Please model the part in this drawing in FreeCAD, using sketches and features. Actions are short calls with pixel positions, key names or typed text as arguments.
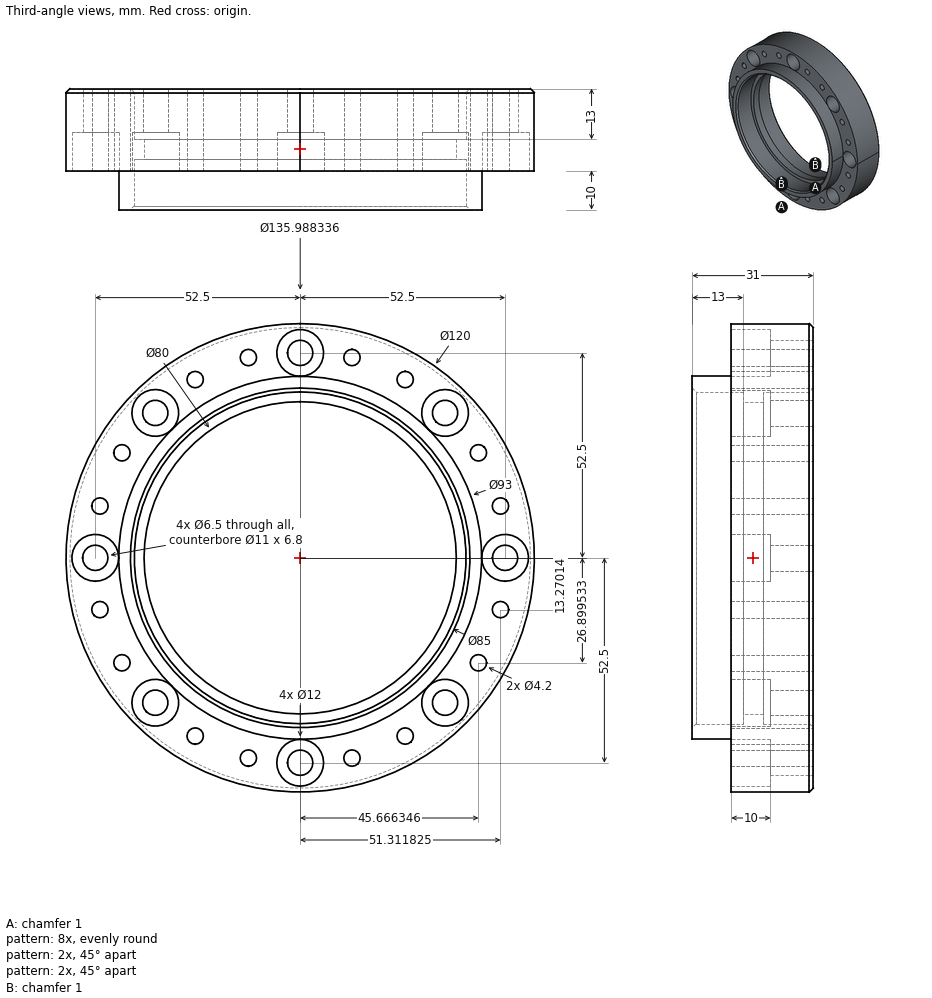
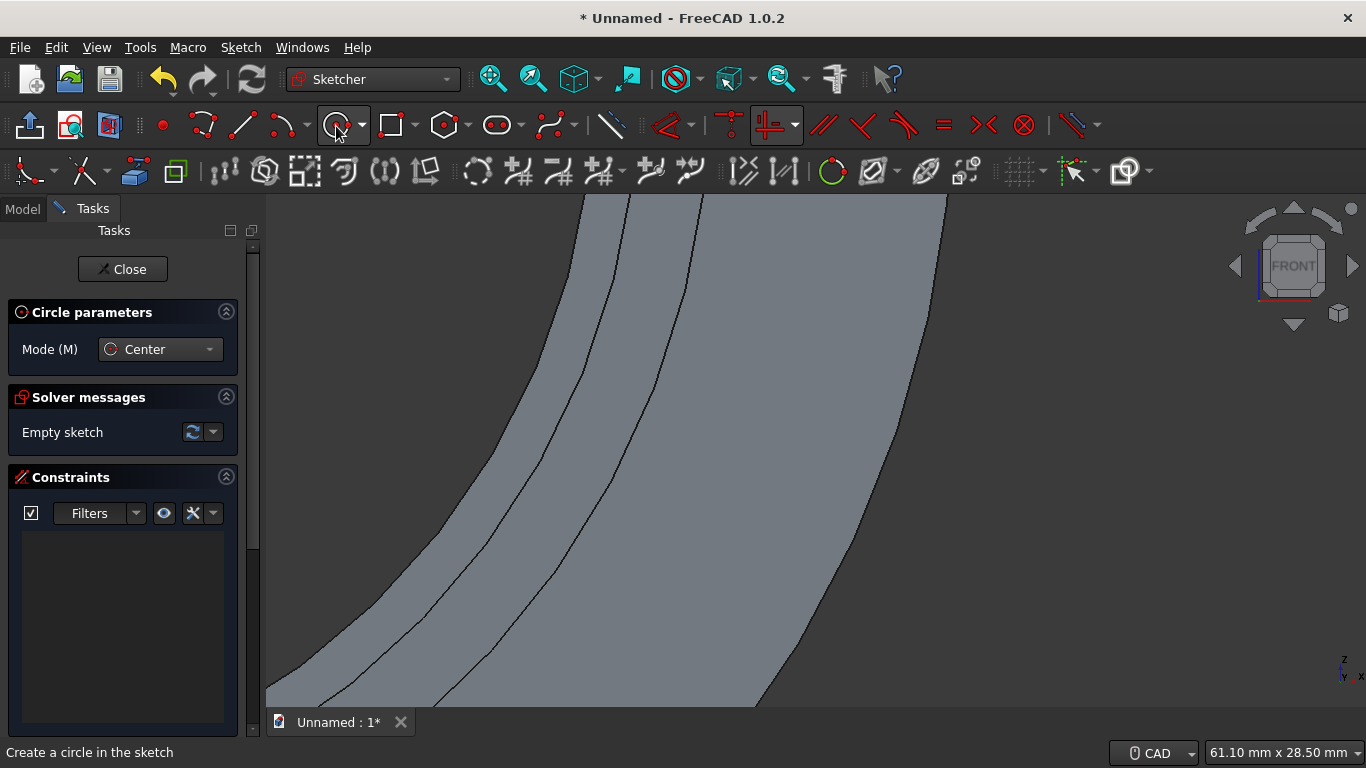
click(695, 570)
move(722, 544)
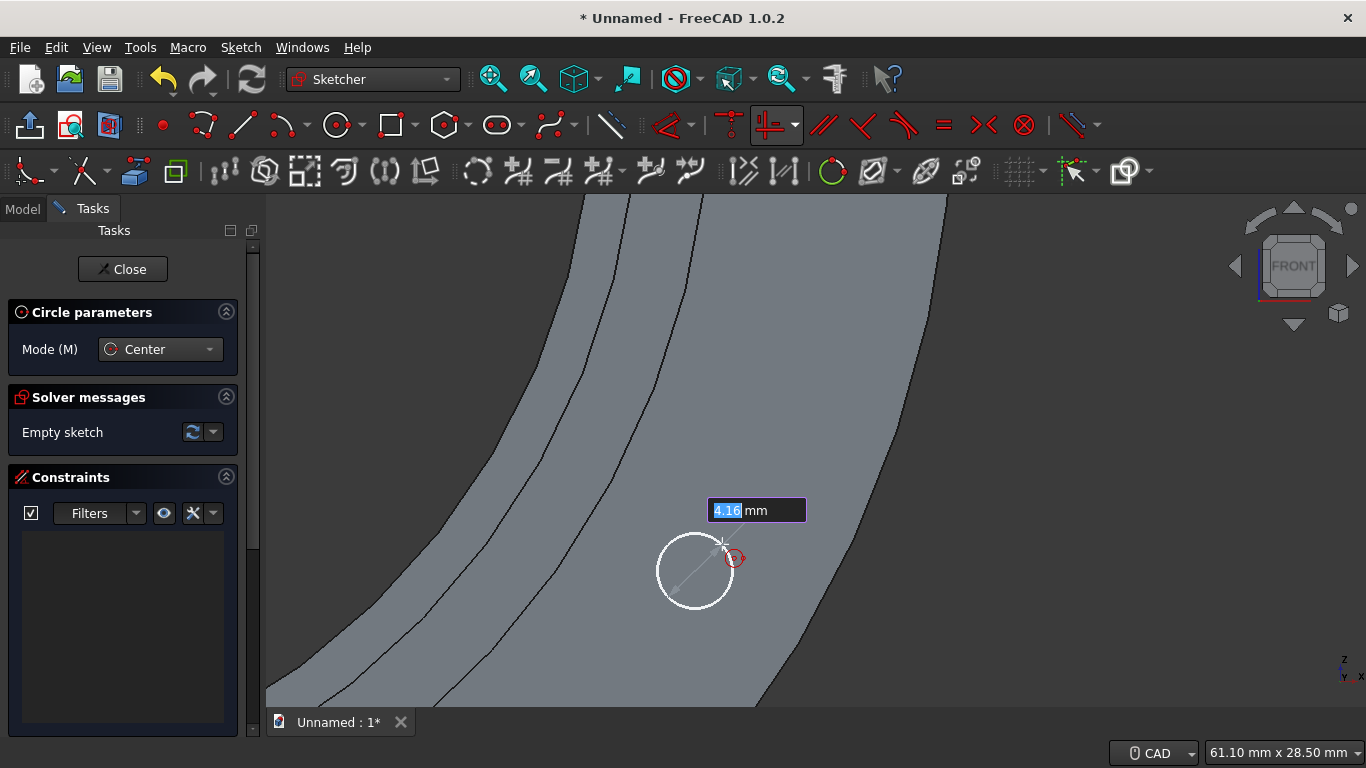
text(4.2)
key(Return)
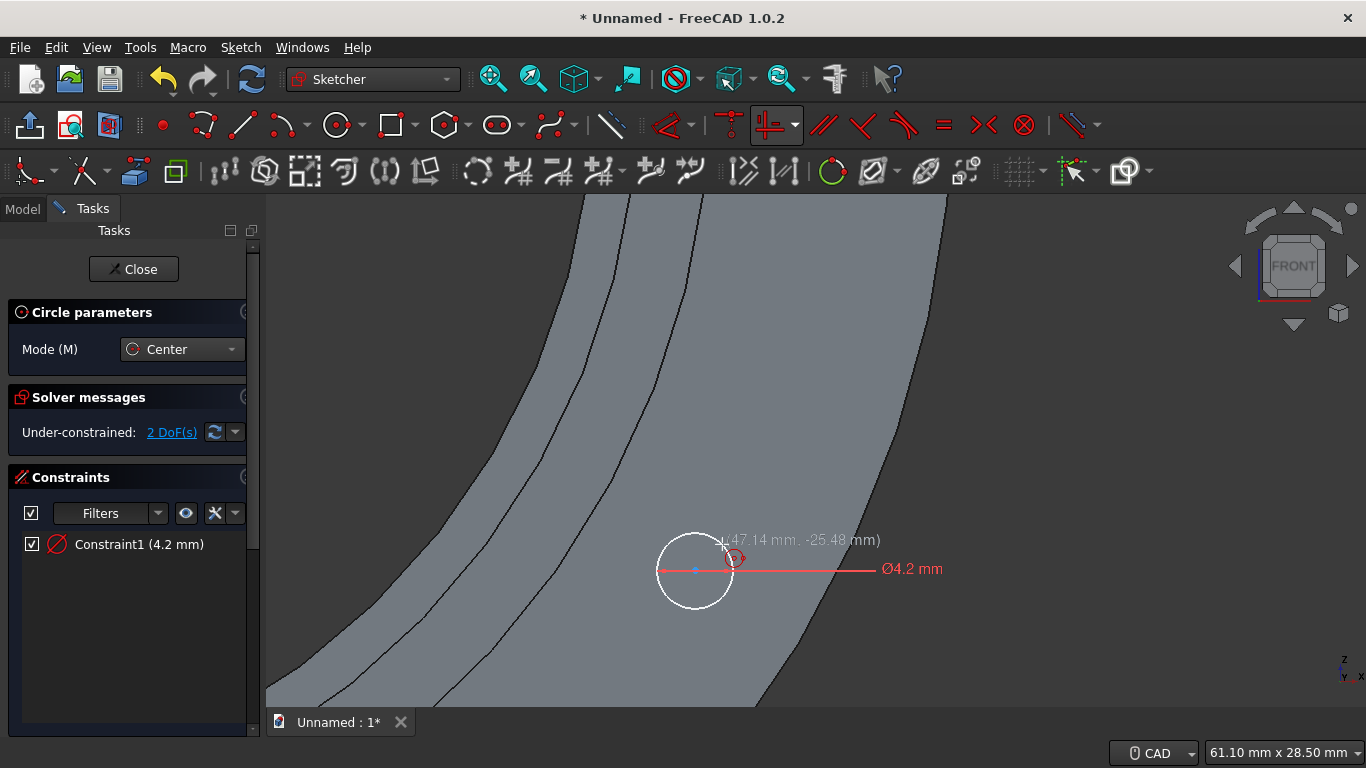
click(797, 325)
move(824, 298)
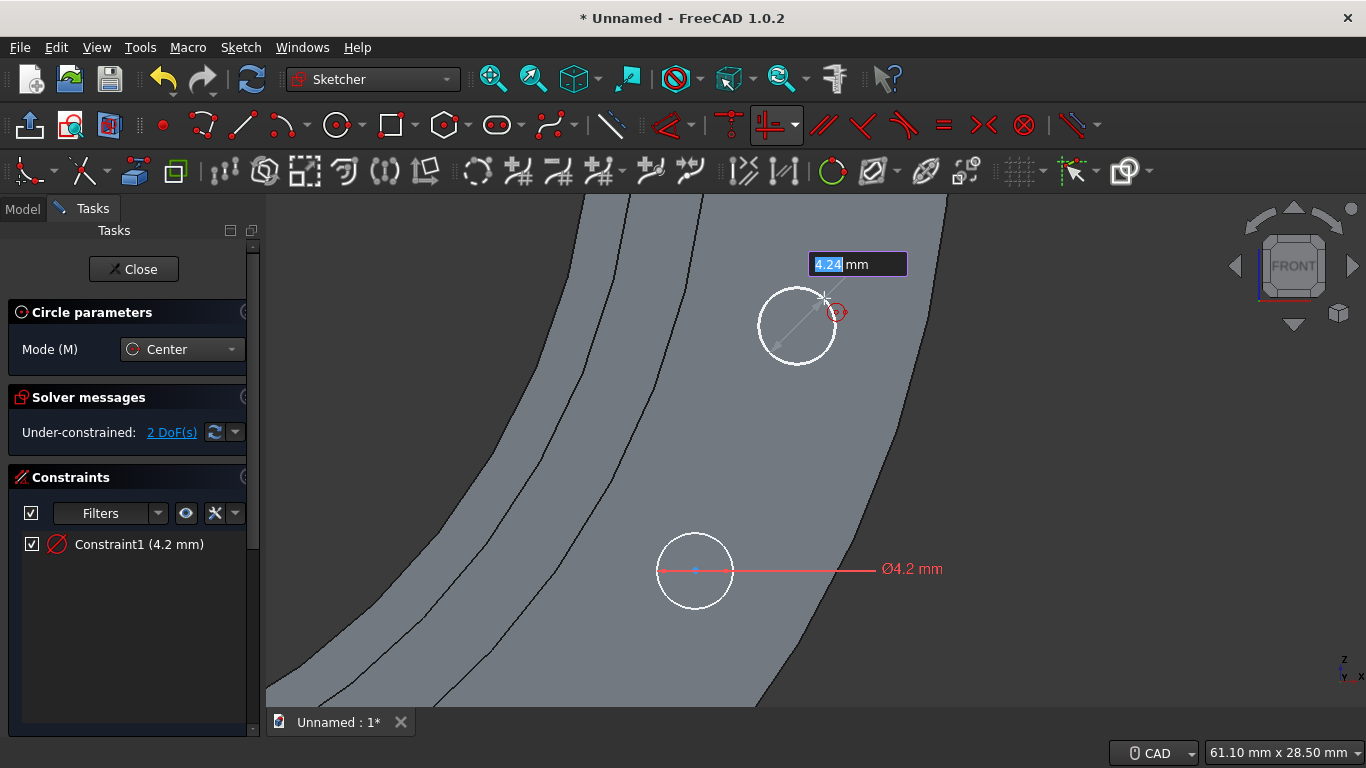
text(4.2)
key(Return)
key(Escape)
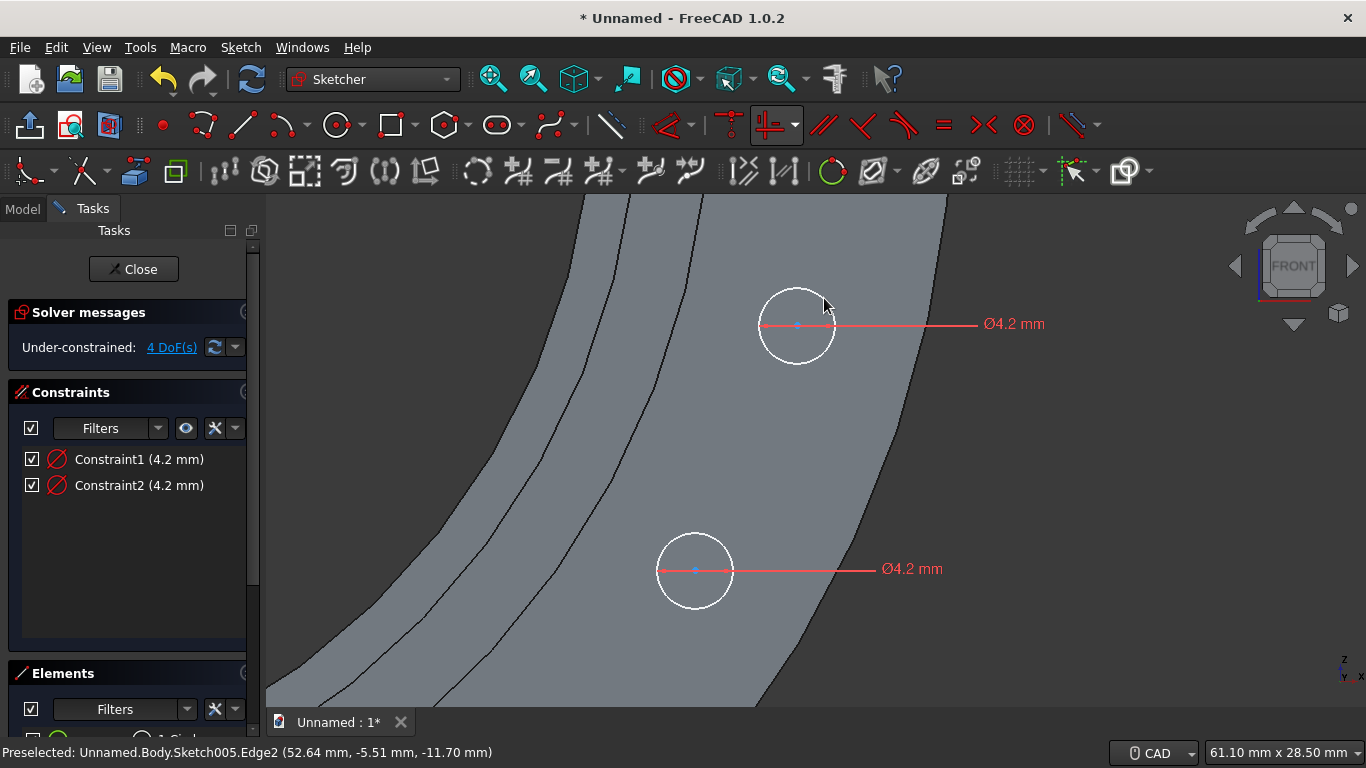
click(666, 126)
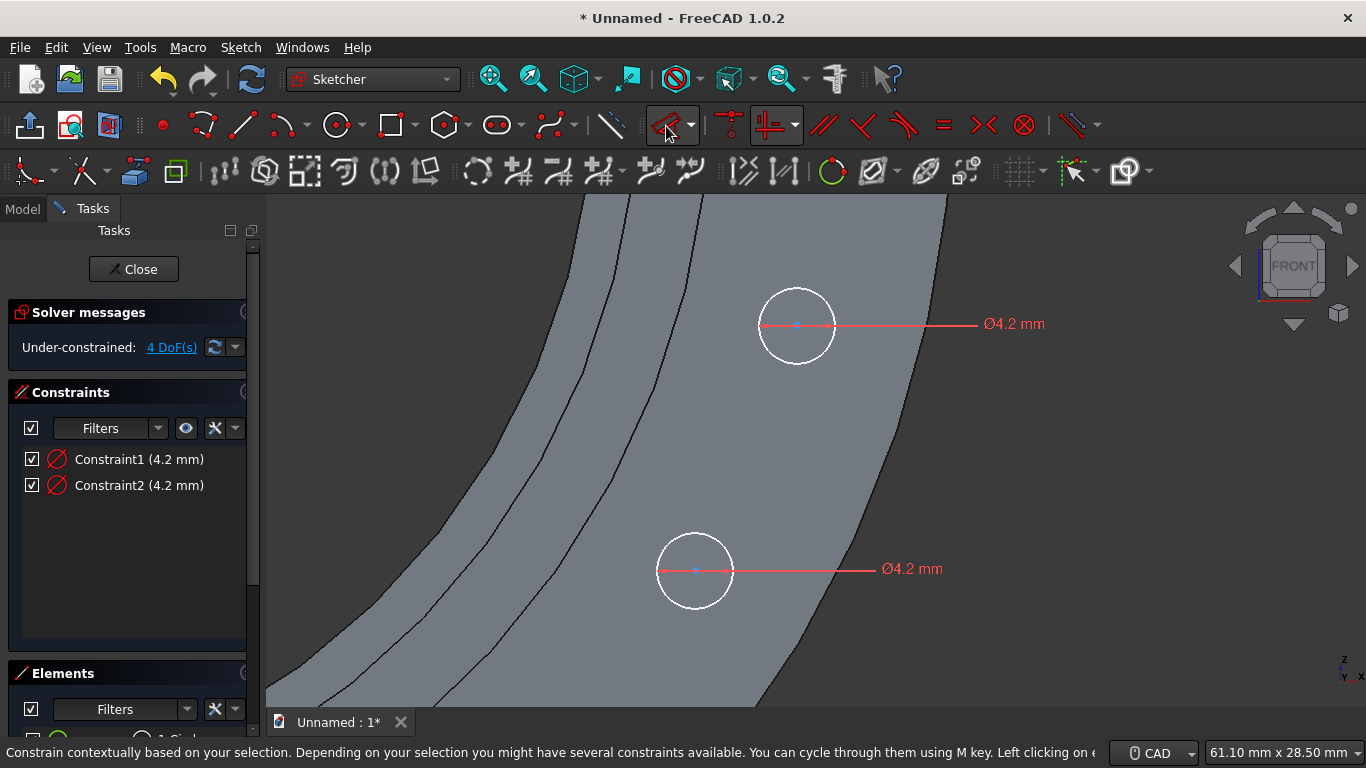
click(797, 326)
click(831, 274)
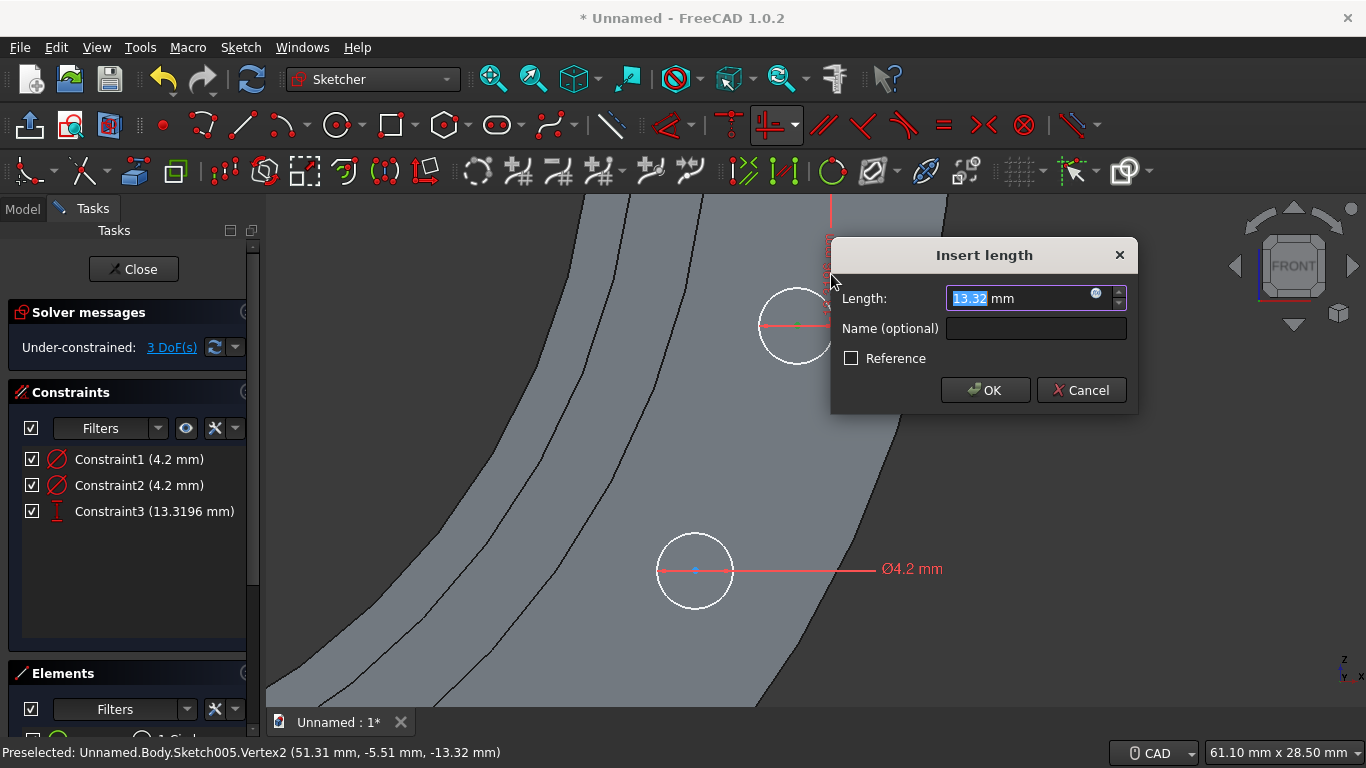
text(13.27014)
key(Return)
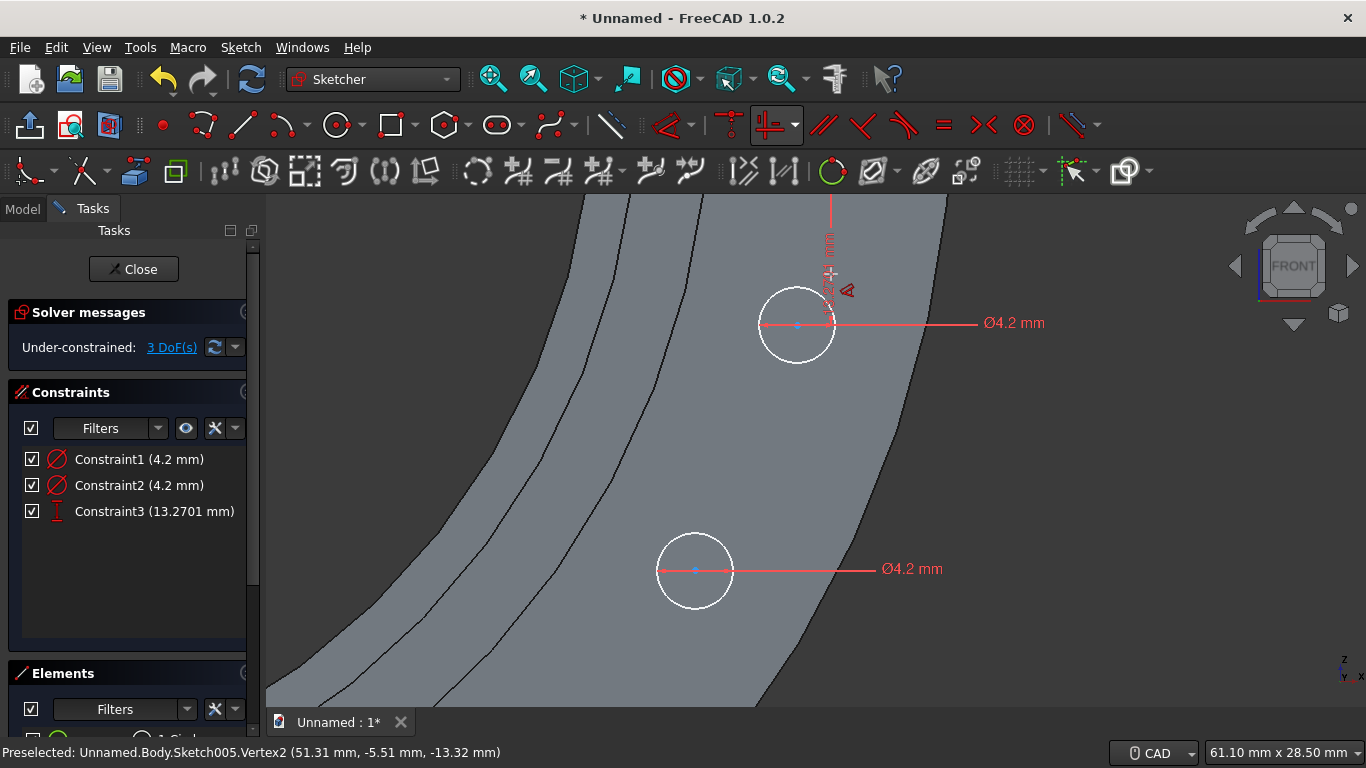
click(695, 571)
click(495, 605)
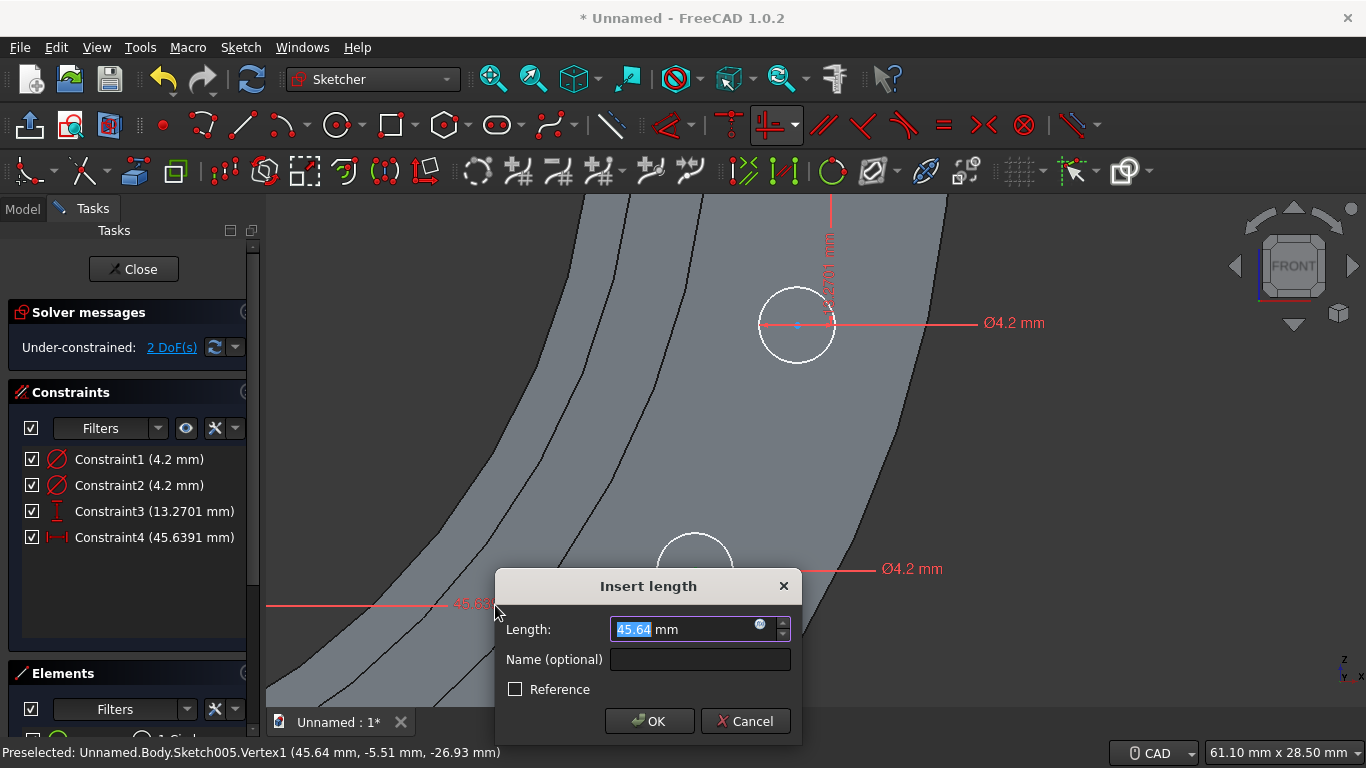
text(45.666346)
key(Return)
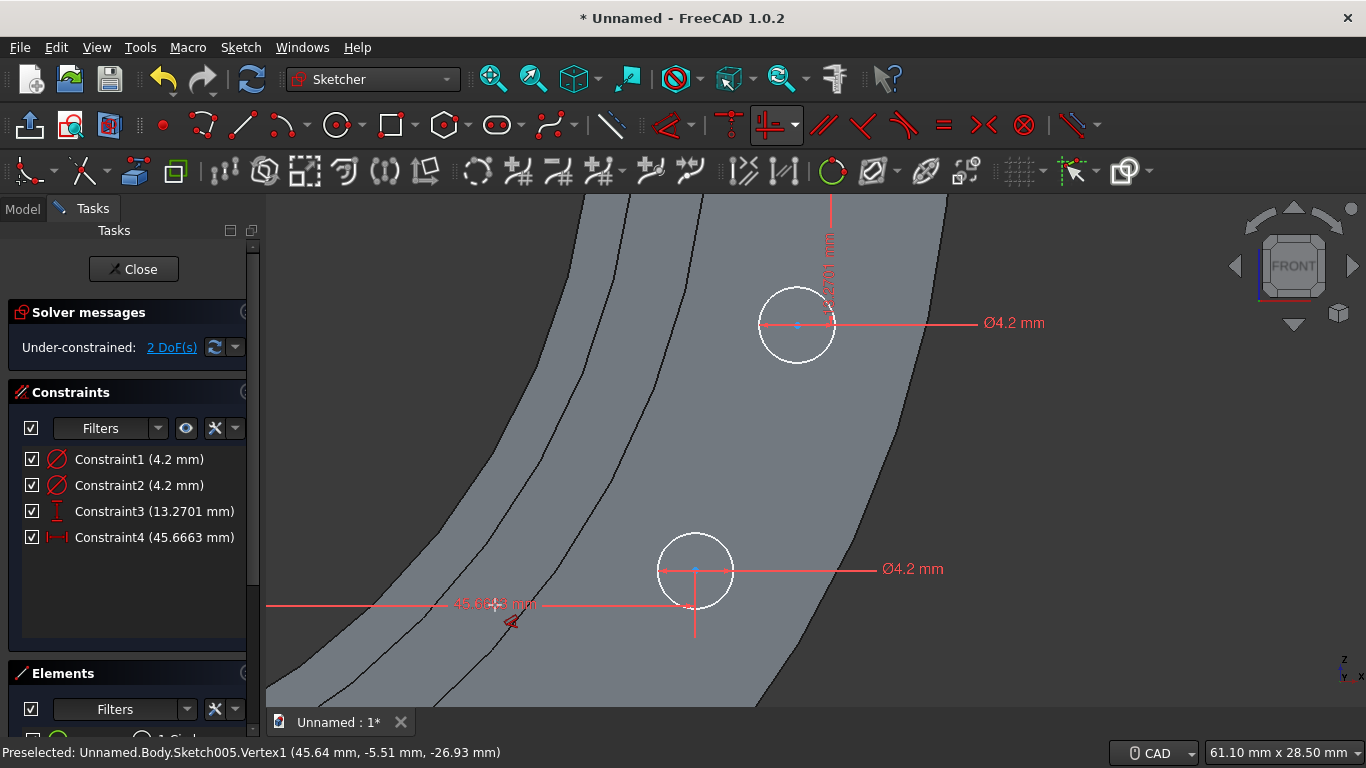
click(695, 571)
click(729, 397)